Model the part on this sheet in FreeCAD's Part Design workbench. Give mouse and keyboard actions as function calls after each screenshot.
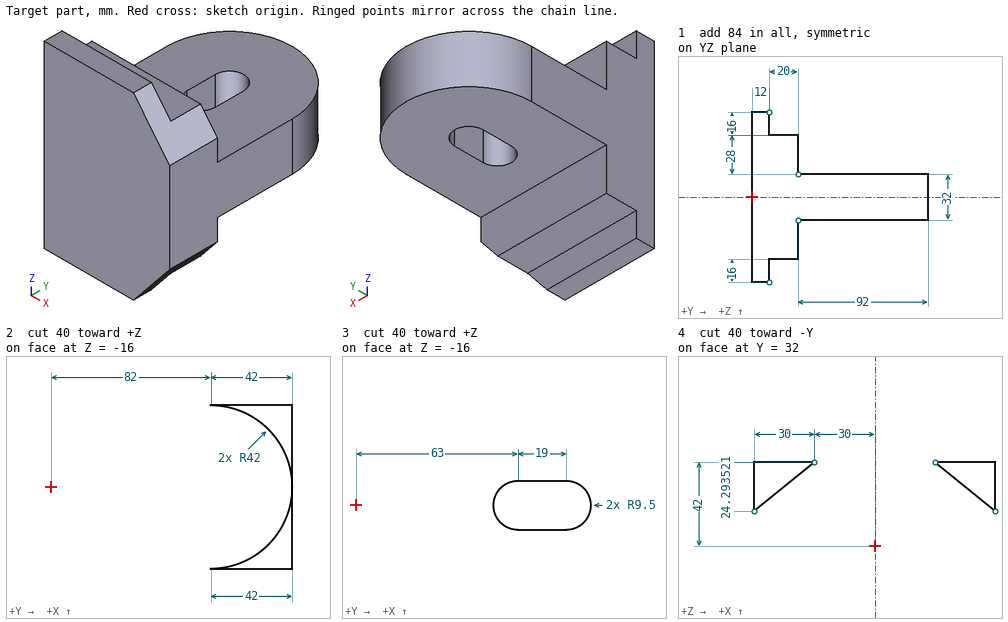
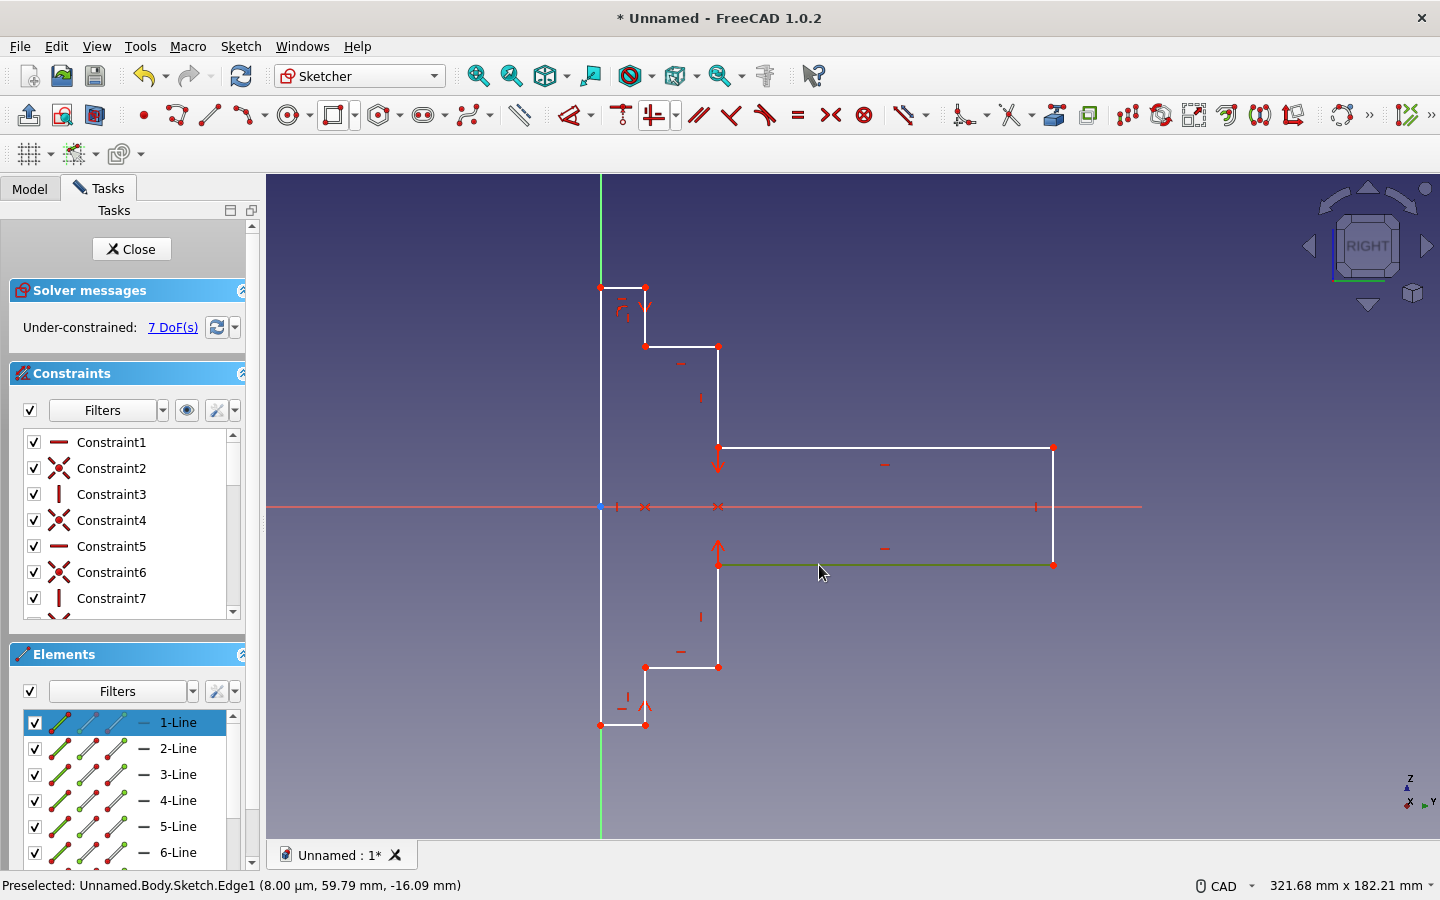
key(l)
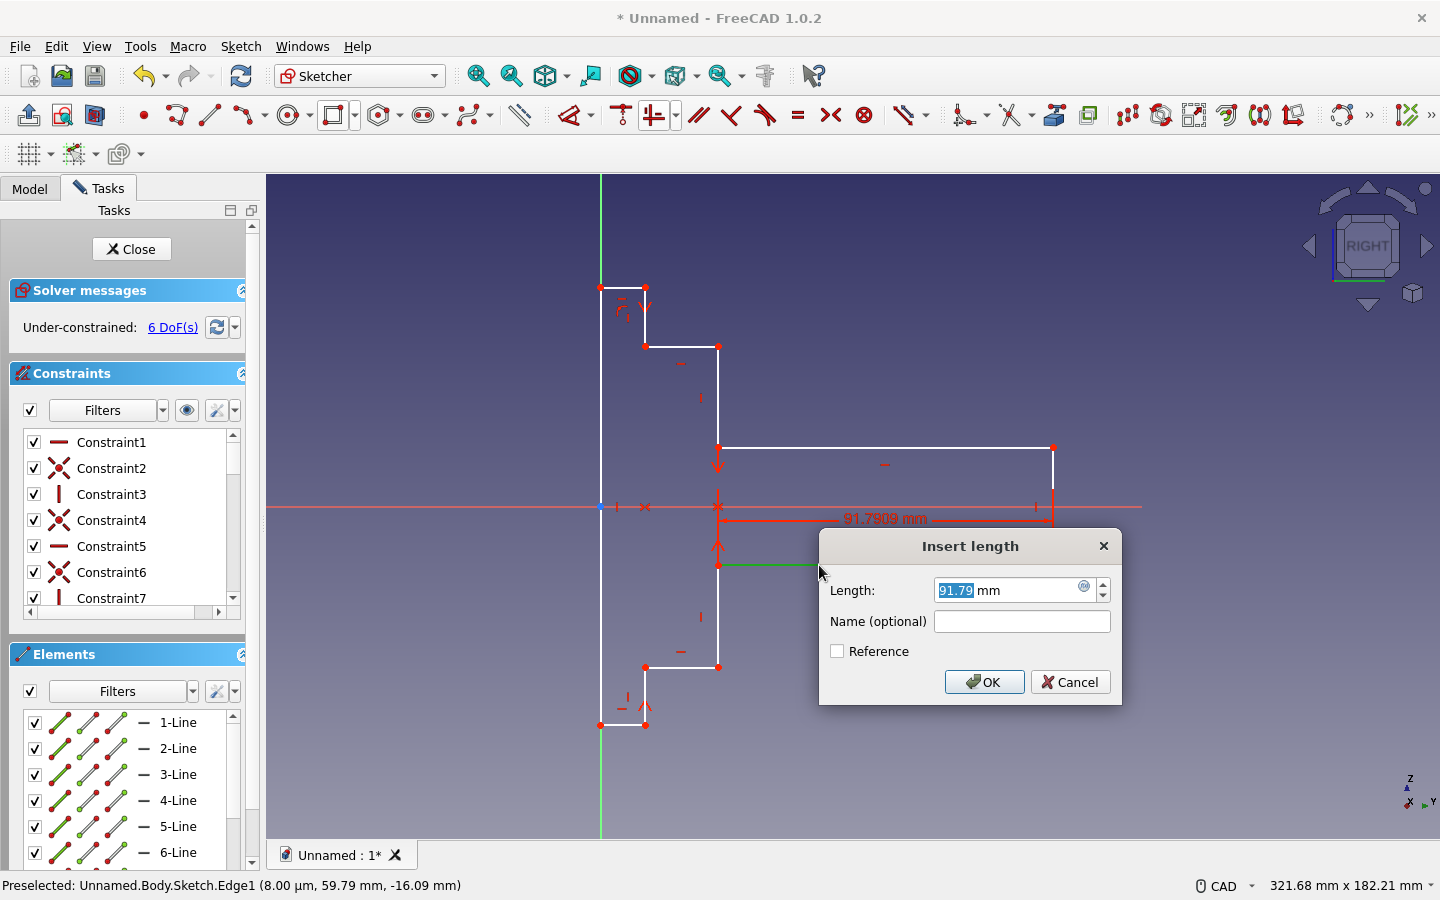
text(92)
key(Return)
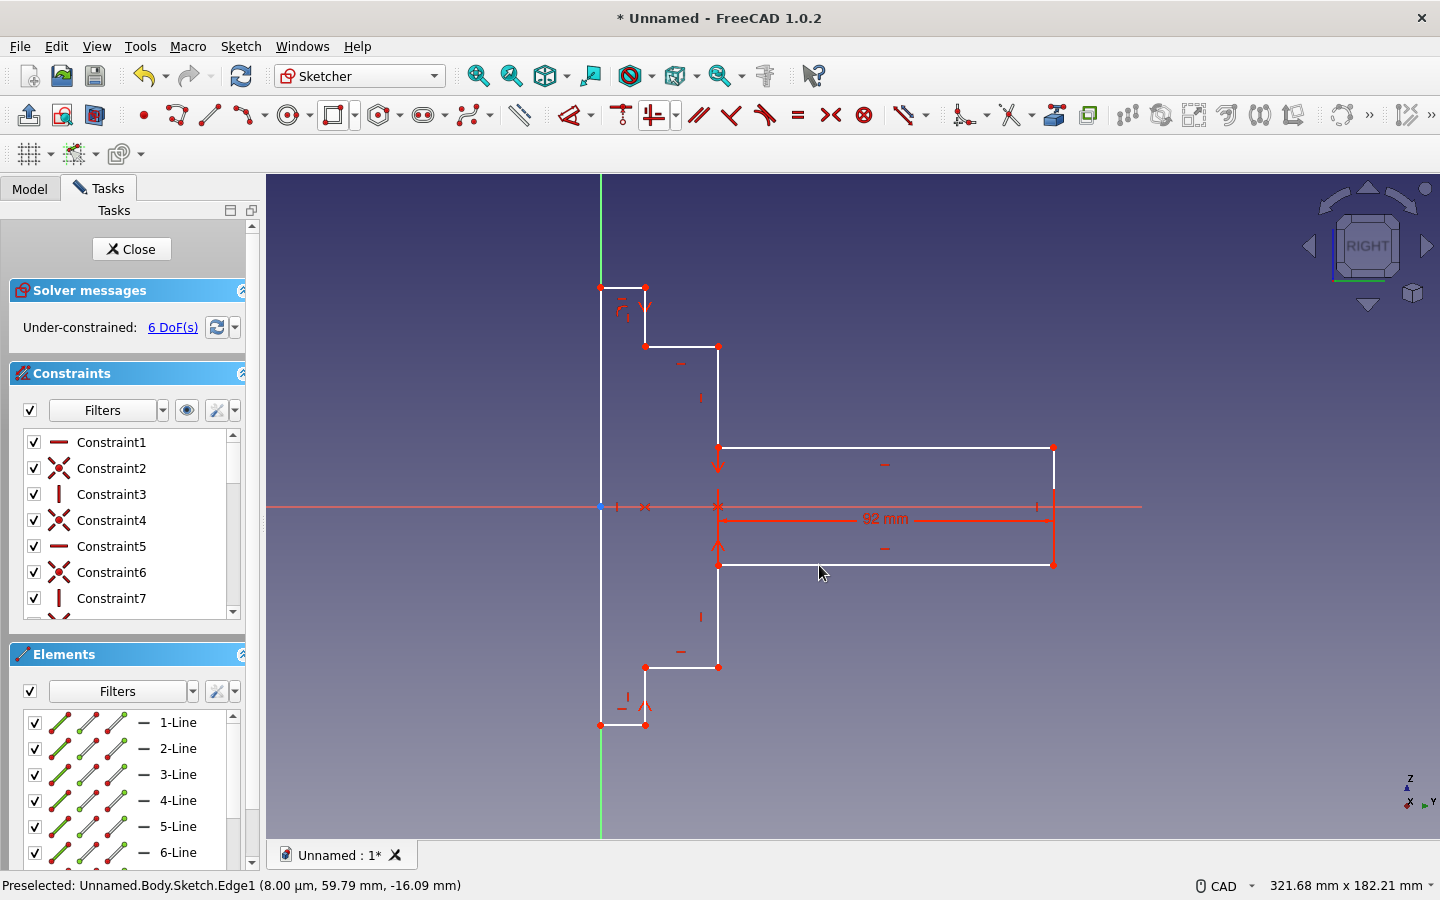
click(1054, 530)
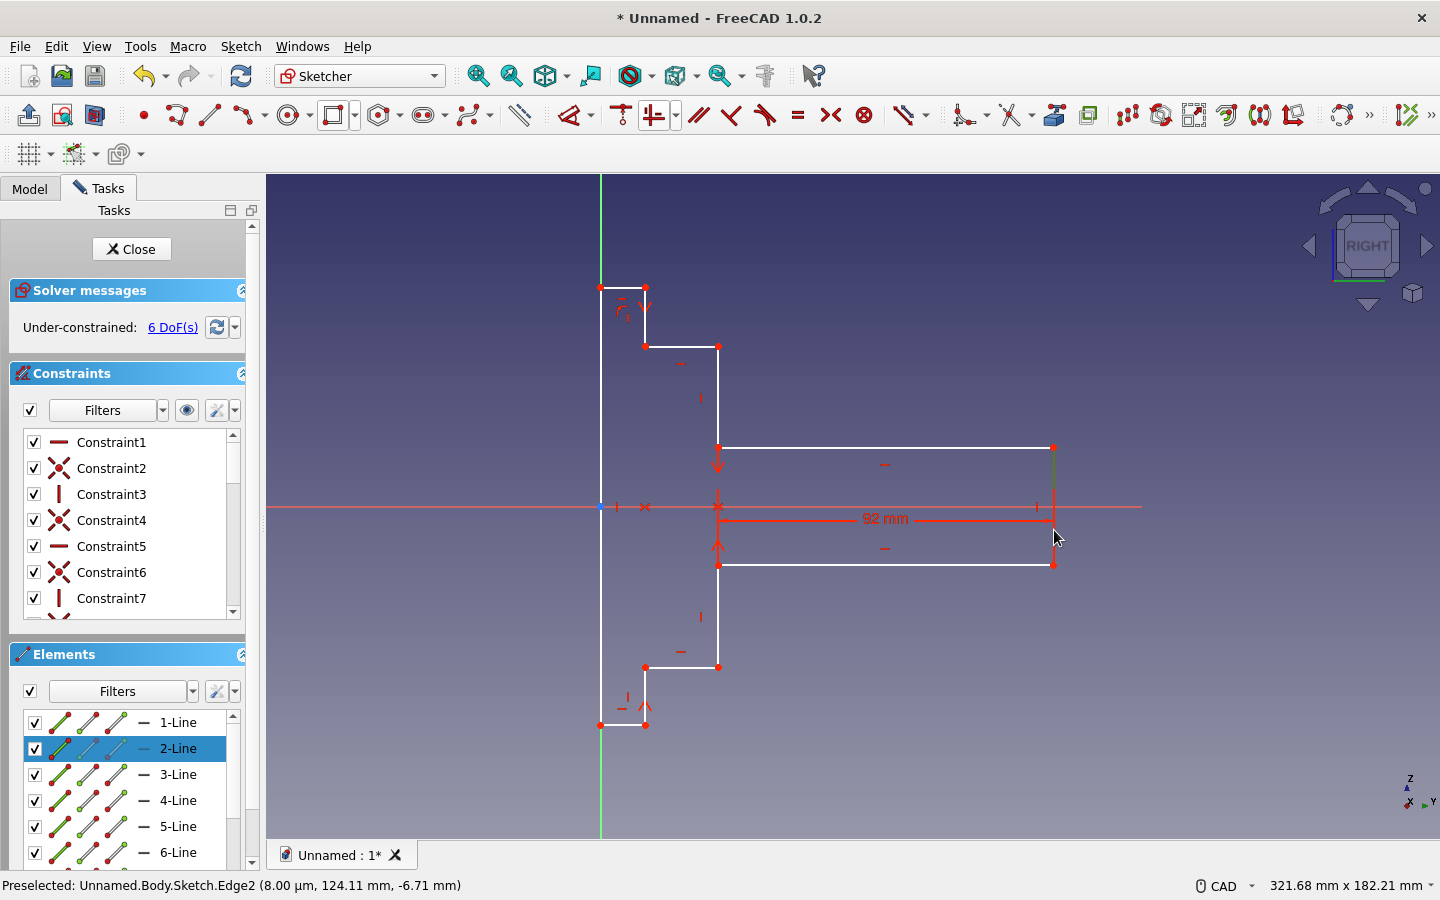
key(i)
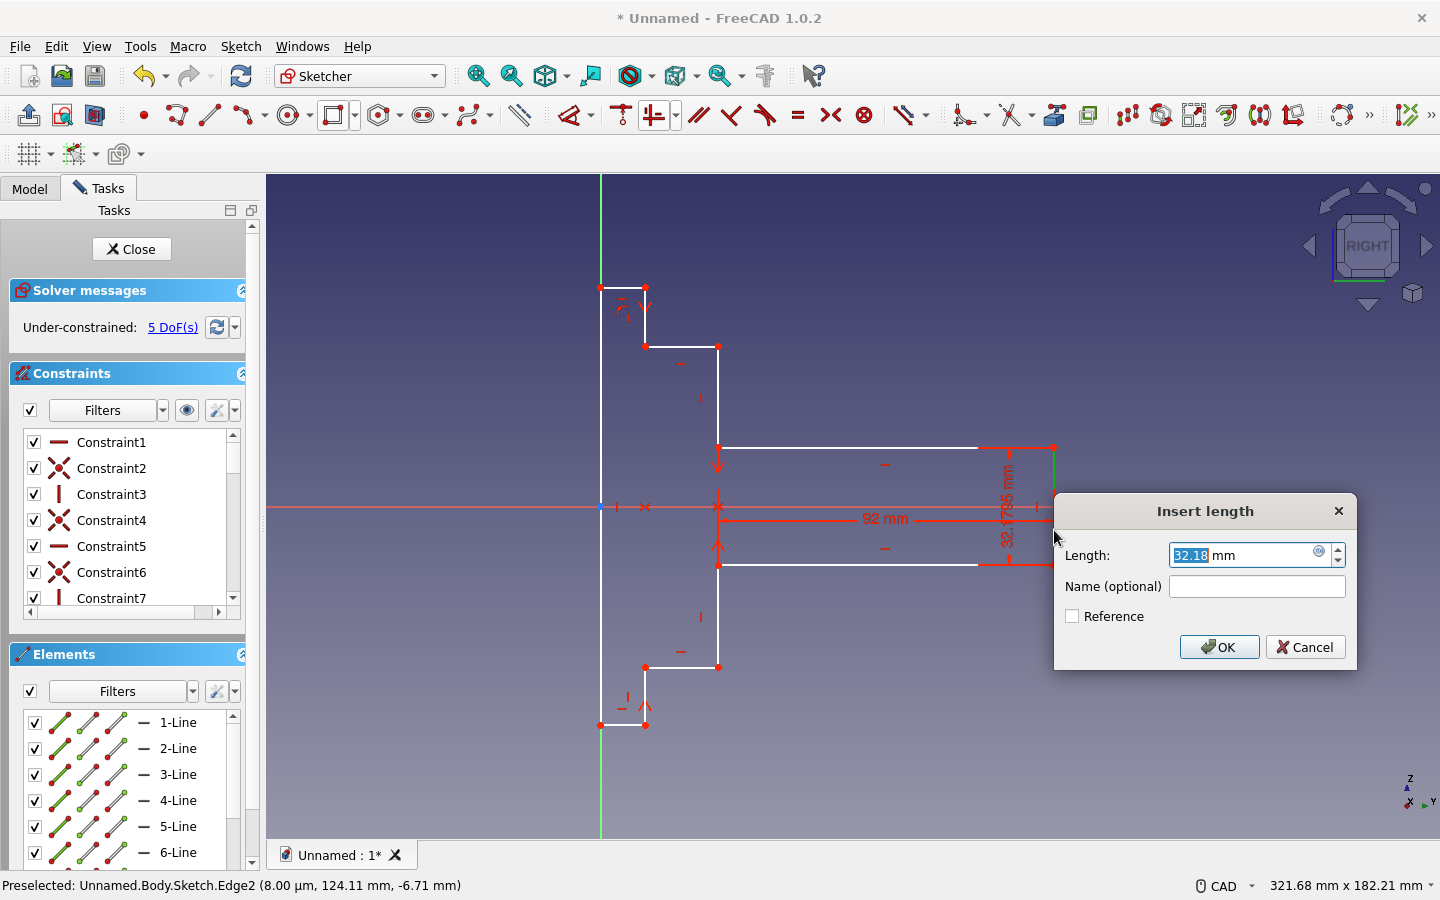
text(32)
key(Return)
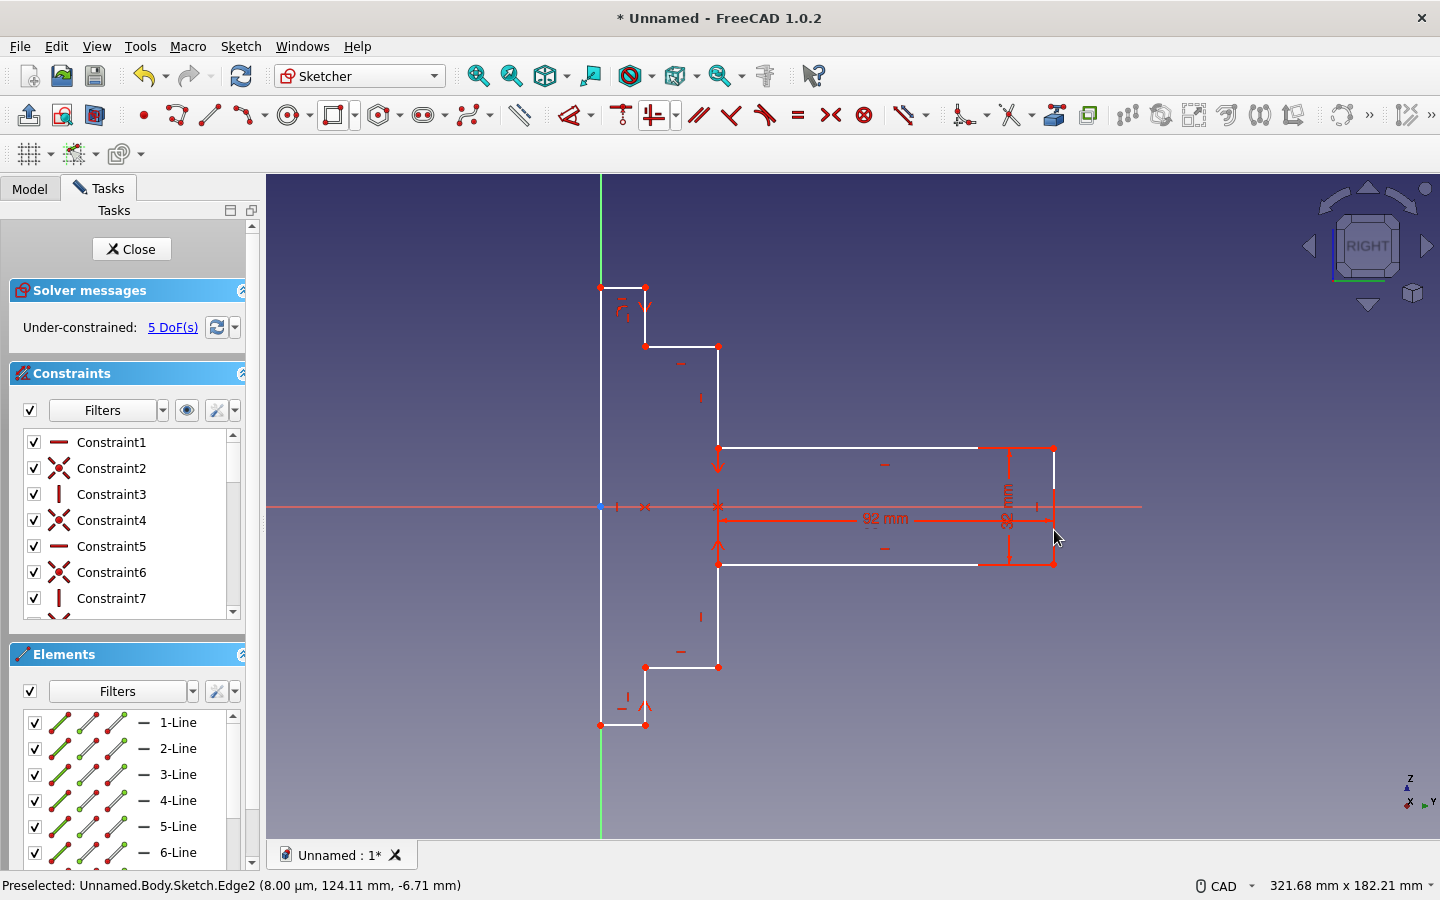
click(718, 418)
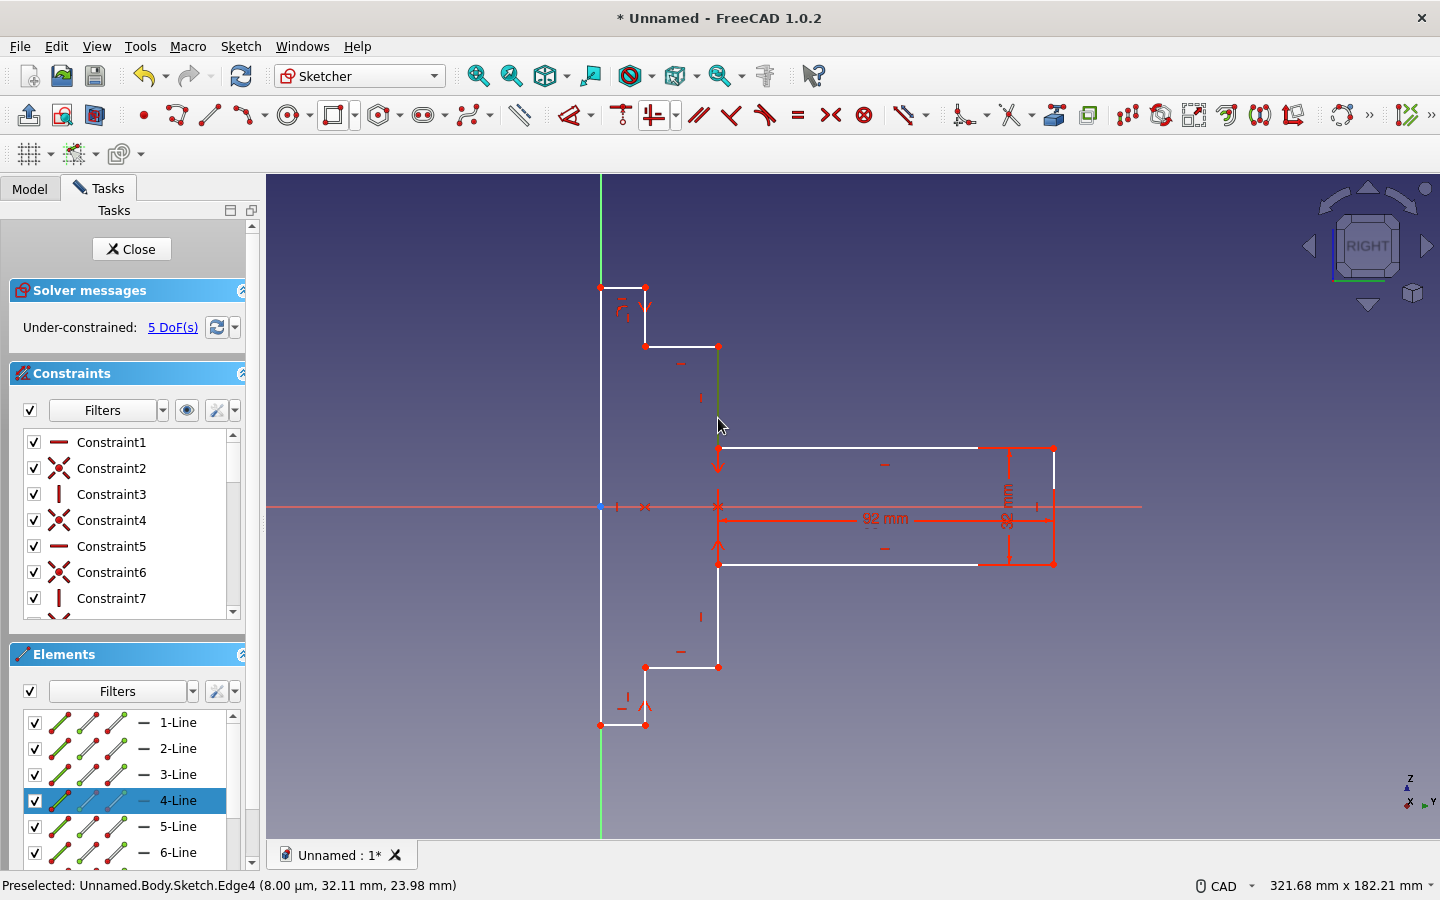
key(i)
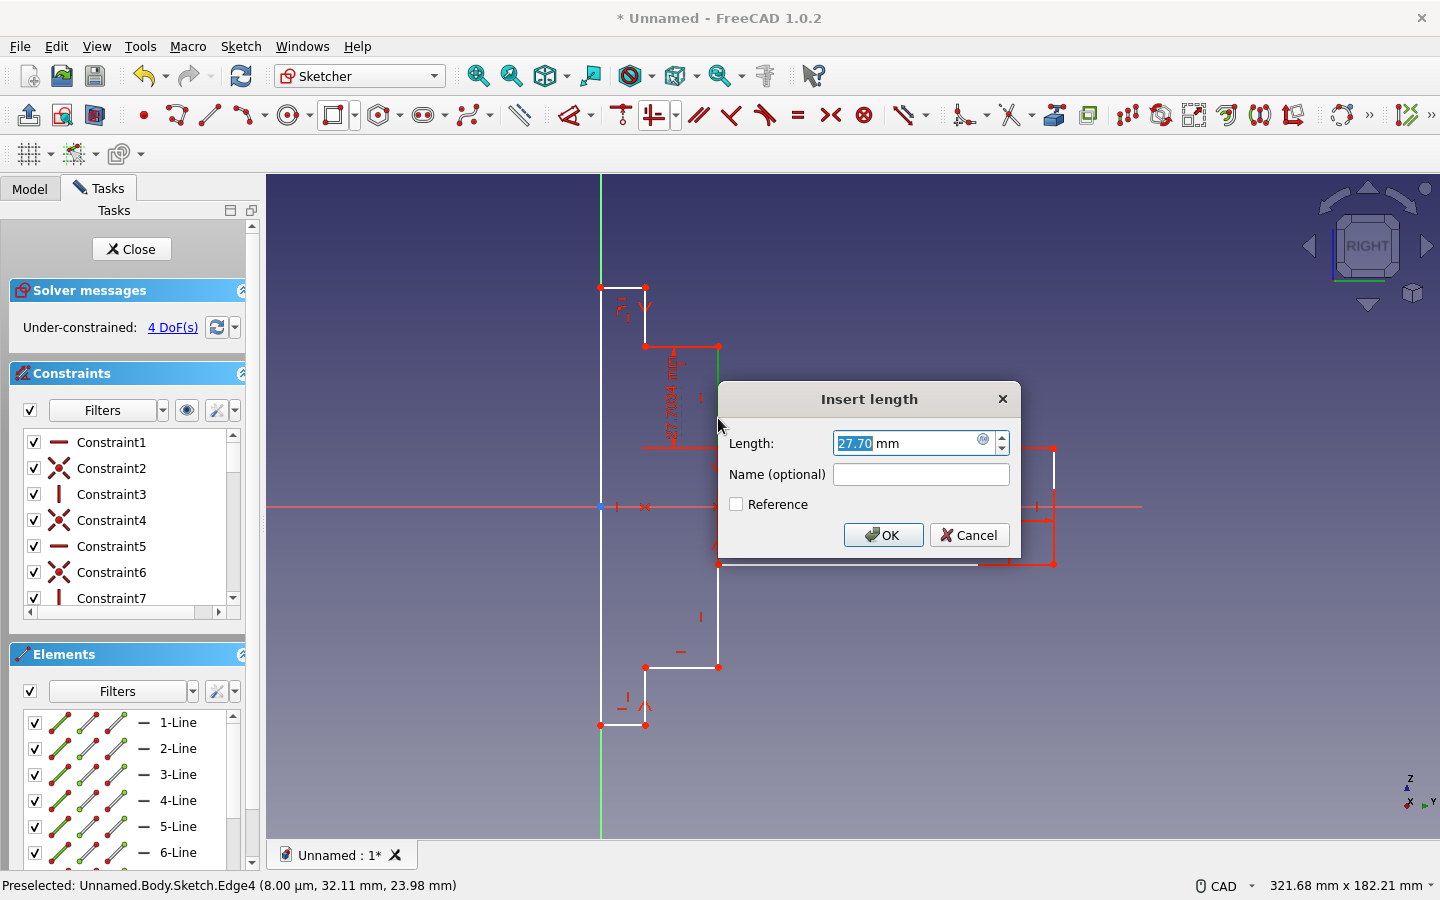
text(28)
key(Return)